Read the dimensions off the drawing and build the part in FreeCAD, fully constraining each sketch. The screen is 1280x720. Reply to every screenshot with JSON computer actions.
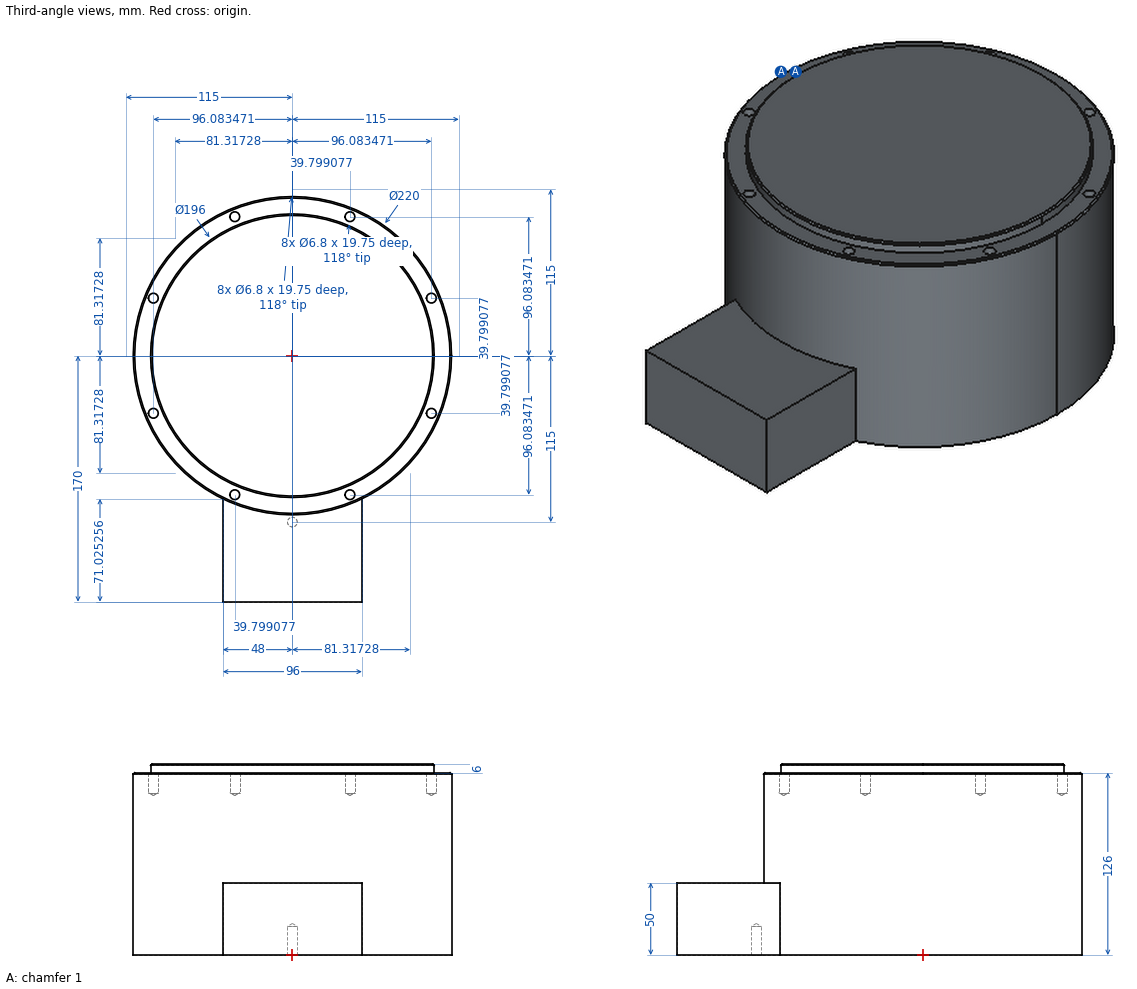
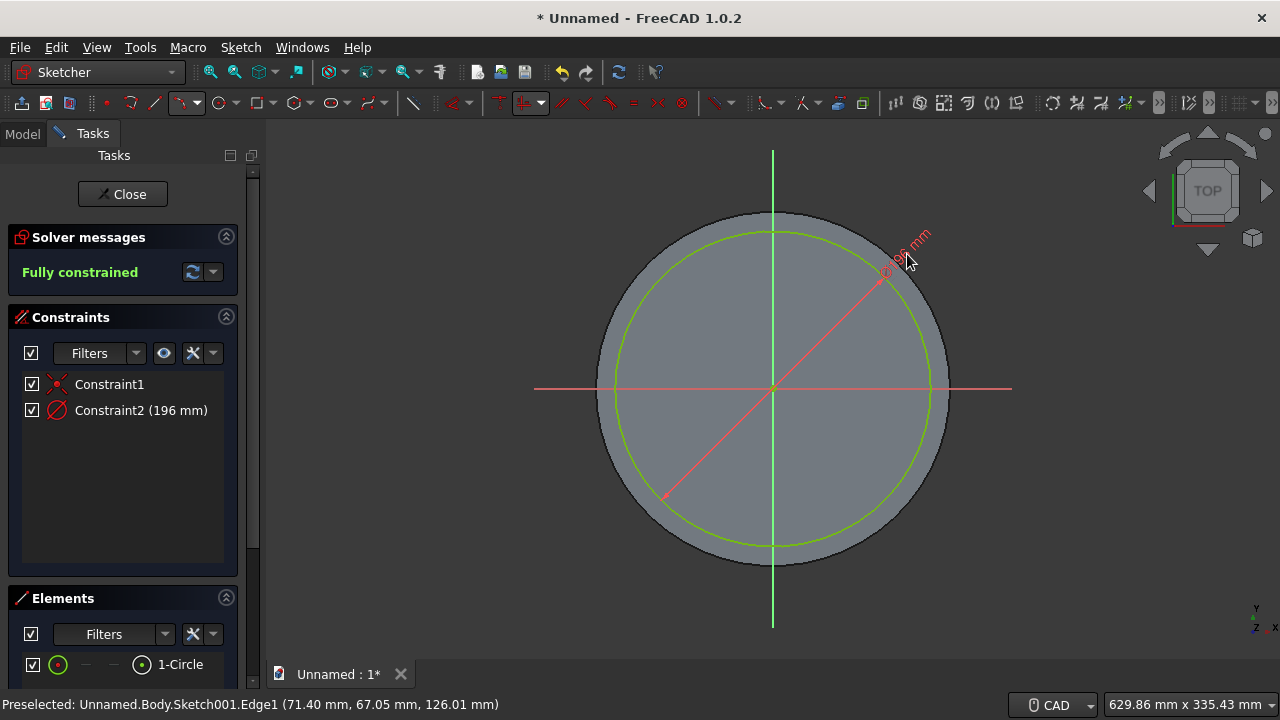
{"action": "left_click", "coordinate": [123, 194]}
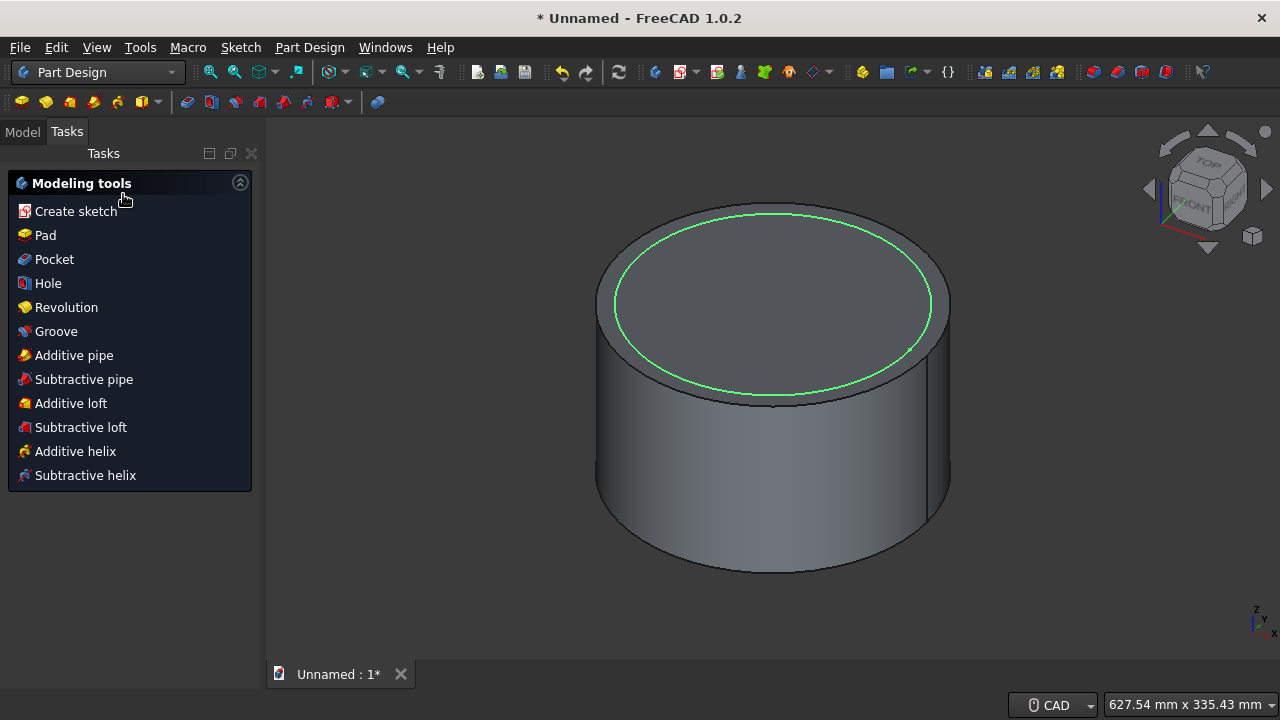
{"action": "left_click", "coordinate": [22, 102]}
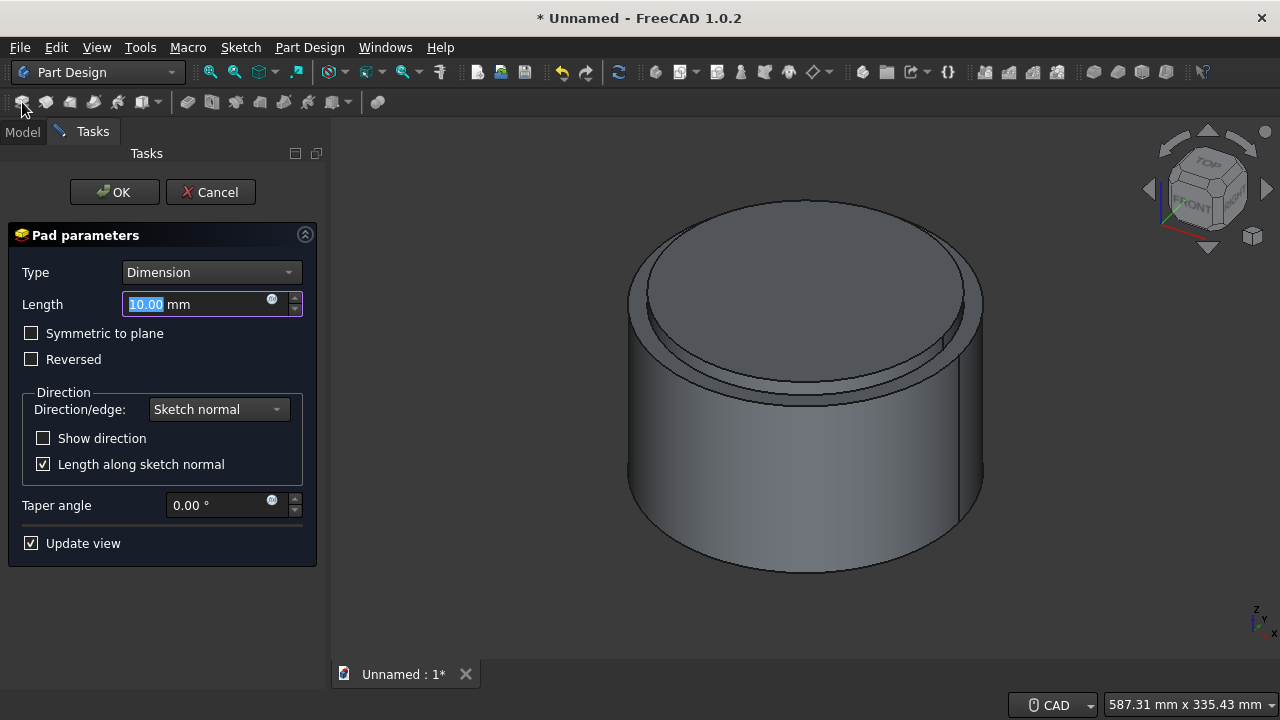
{"action": "type", "text": "6"}
{"action": "key", "text": "Tab"}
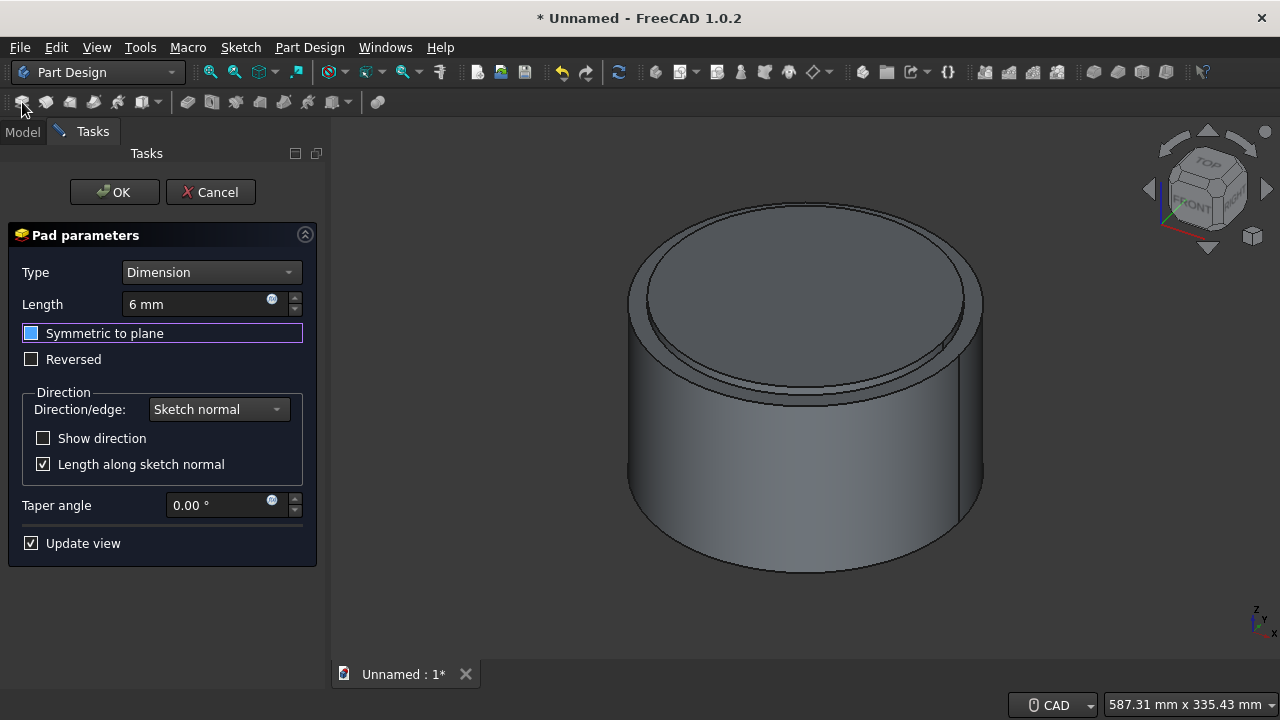
{"action": "left_click", "coordinate": [115, 192]}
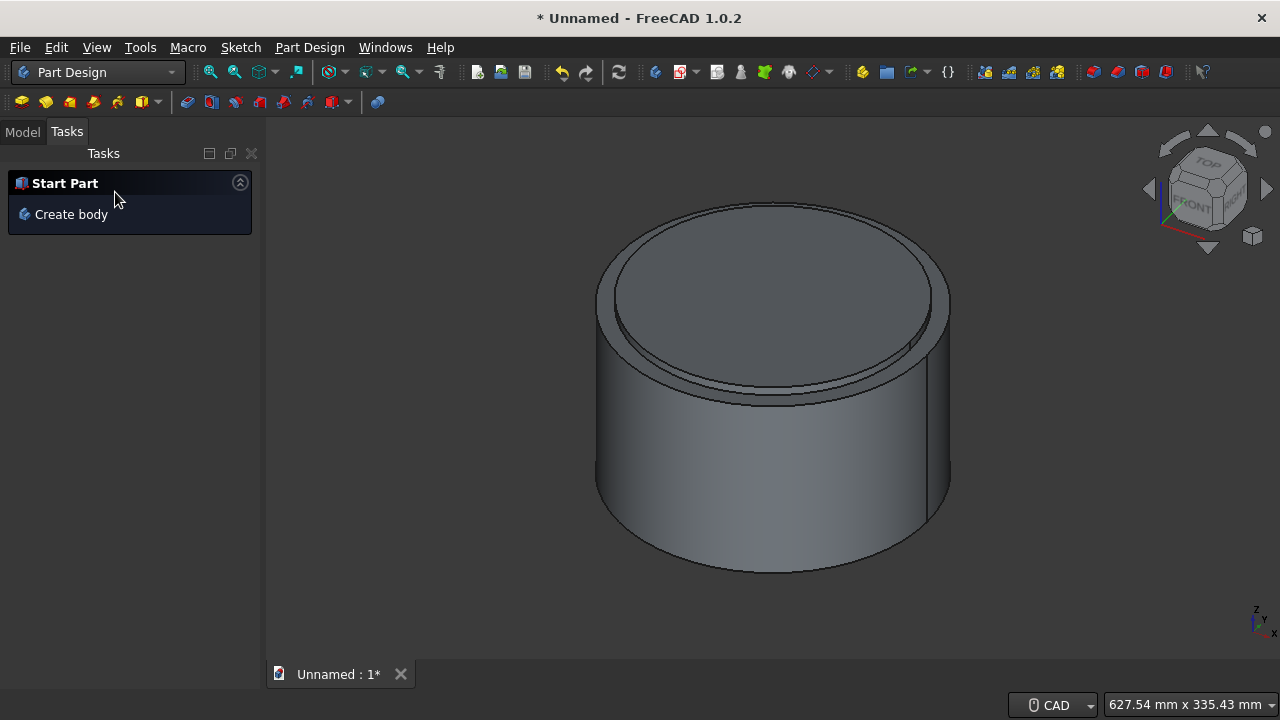
{"action": "key", "text": "5"}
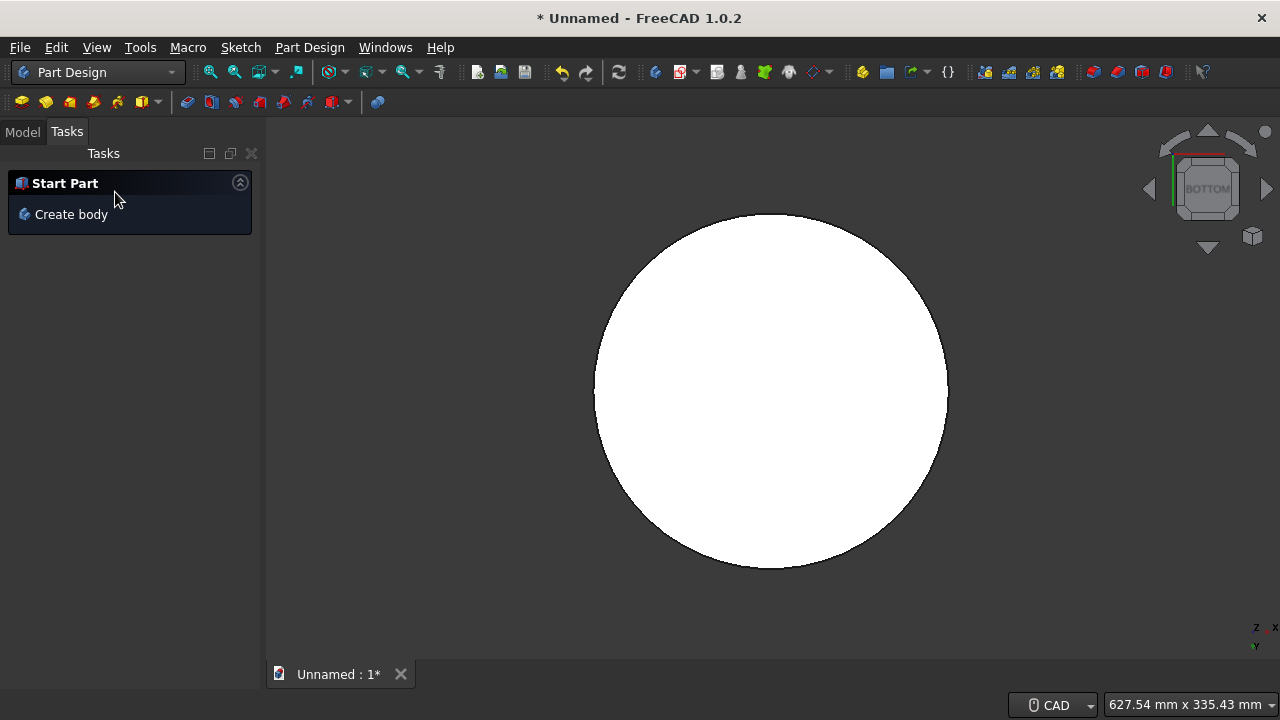
{"action": "left_click", "coordinate": [771, 390]}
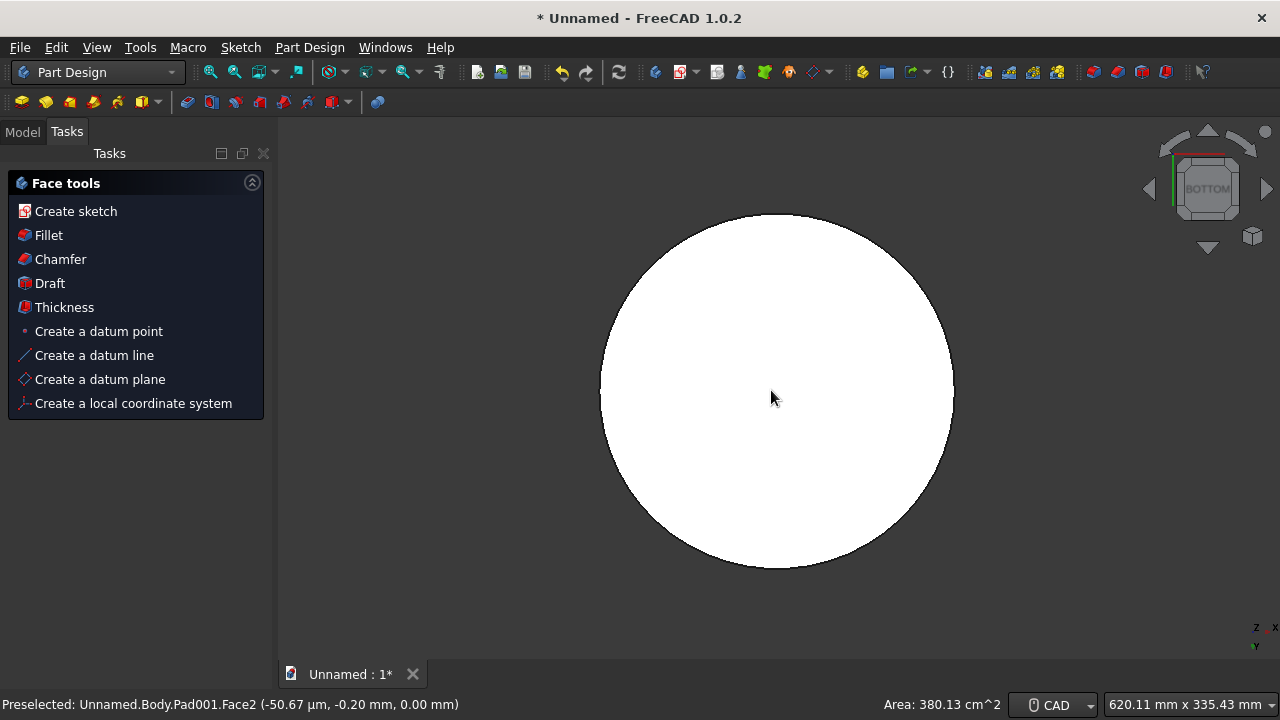
{"action": "left_click", "coordinate": [680, 72]}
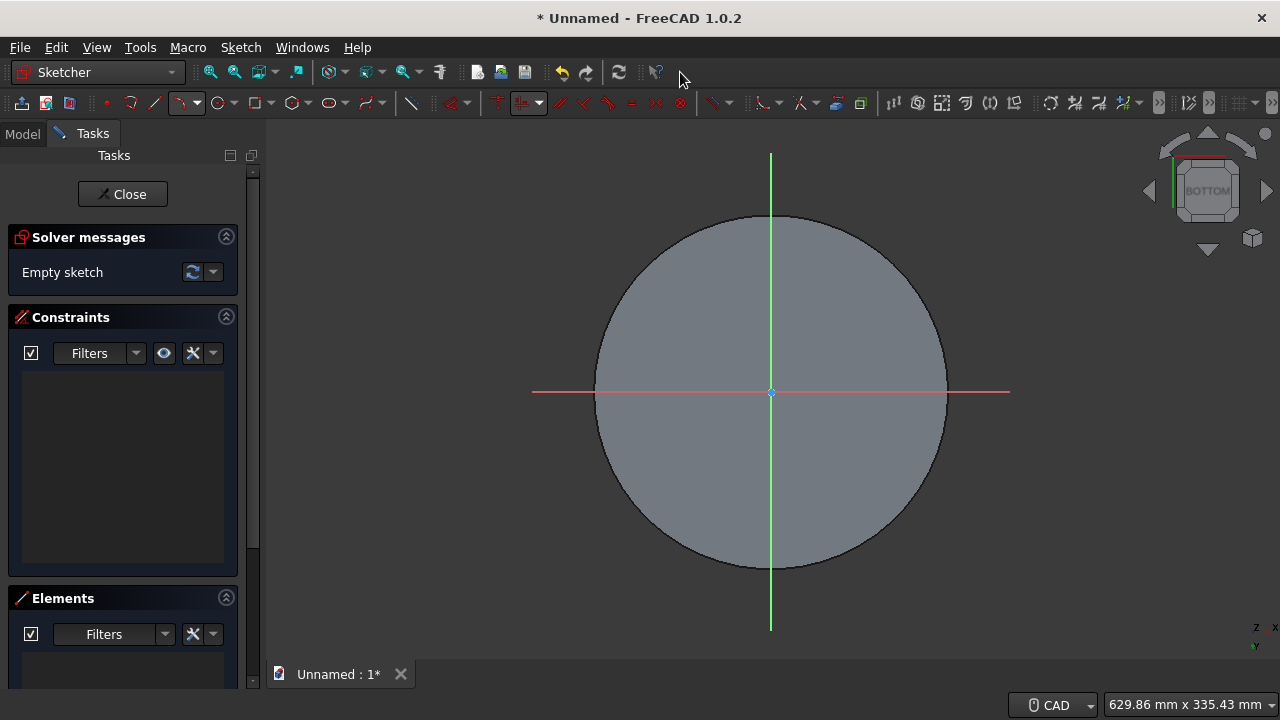
{"action": "scroll", "coordinate": [404, 631], "scroll_direction": "down", "scroll_amount": 1}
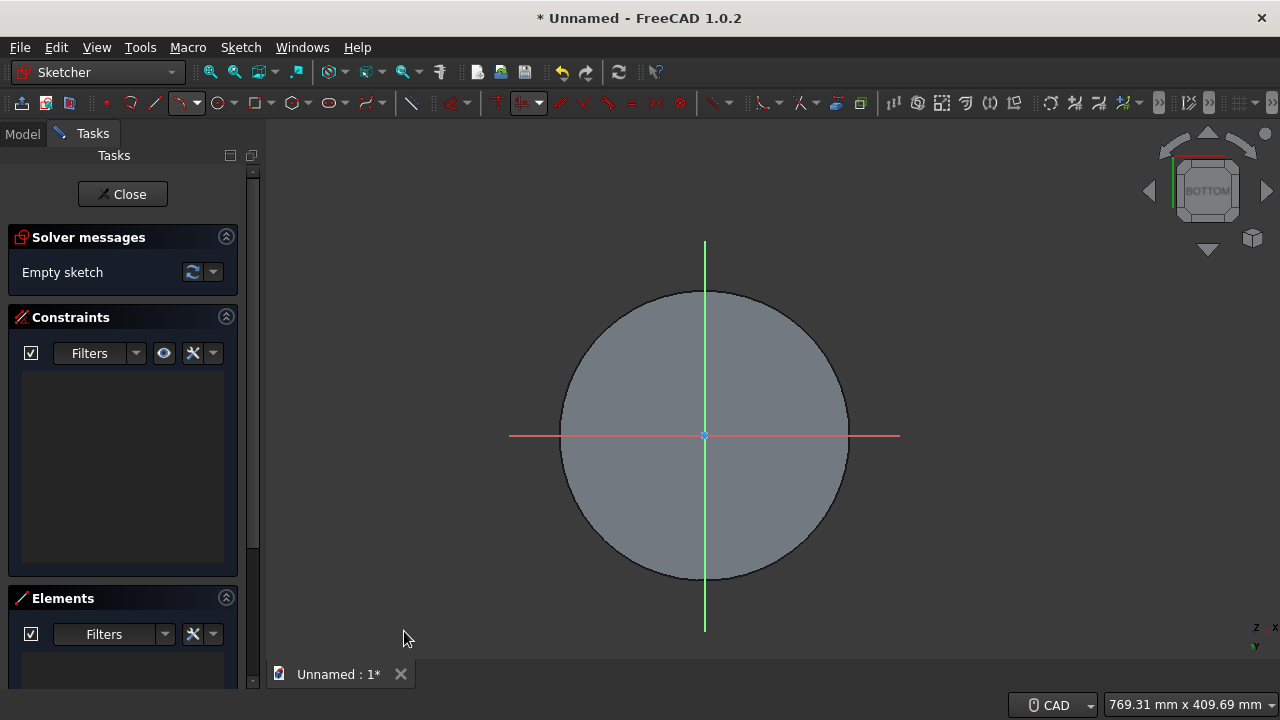
{"action": "scroll", "coordinate": [705, 191], "scroll_direction": "up", "scroll_amount": 2}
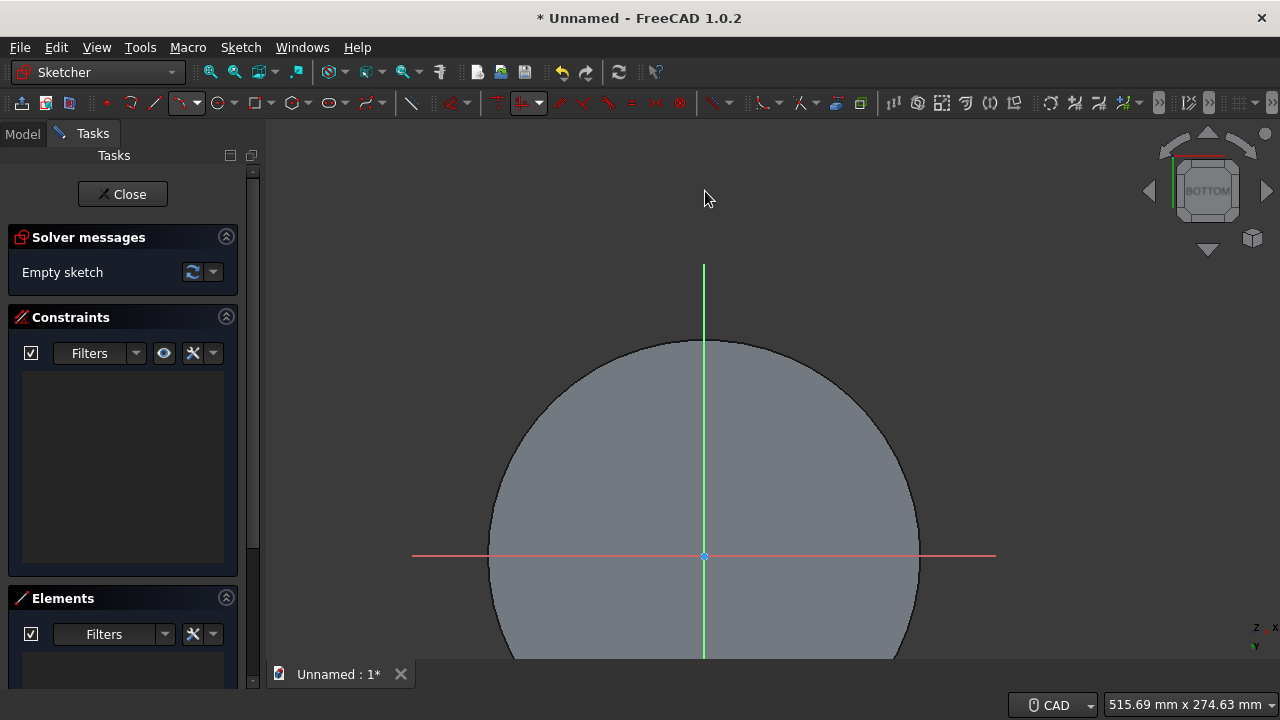
{"action": "left_click", "coordinate": [256, 104]}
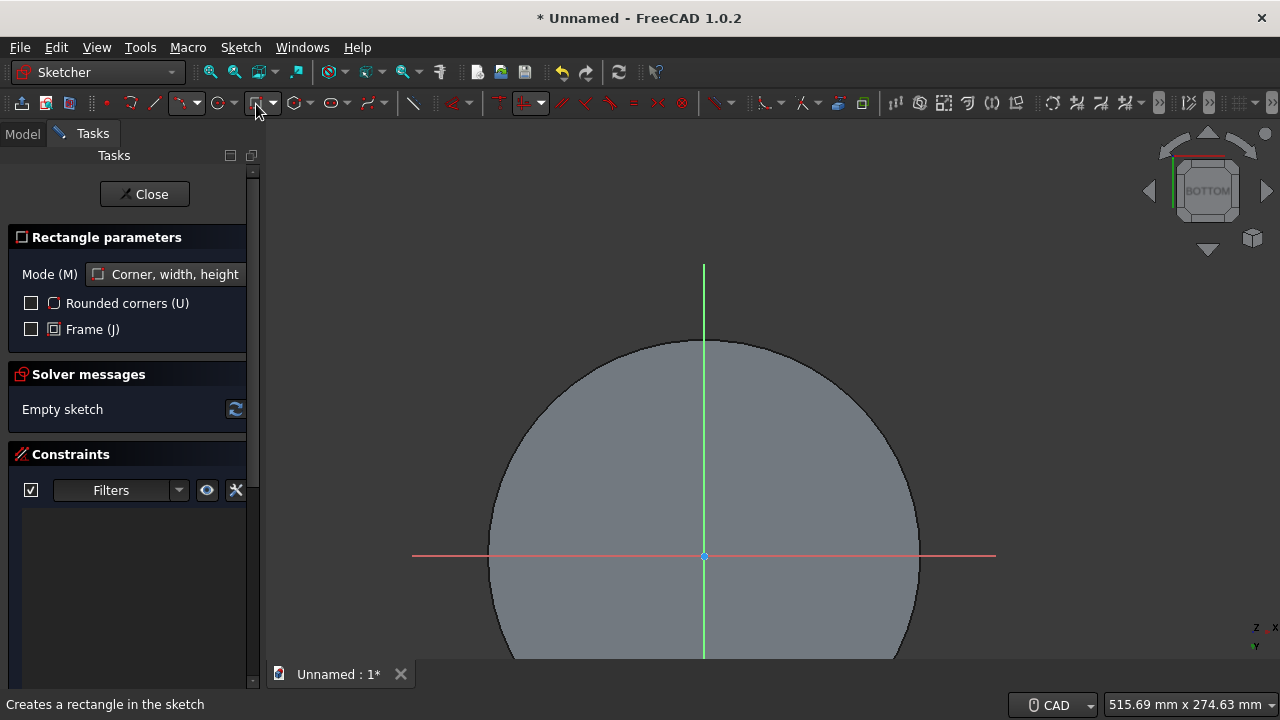
{"action": "left_click", "coordinate": [610, 222]}
{"action": "left_click", "coordinate": [799, 361]}
{"action": "key", "text": "Escape"}